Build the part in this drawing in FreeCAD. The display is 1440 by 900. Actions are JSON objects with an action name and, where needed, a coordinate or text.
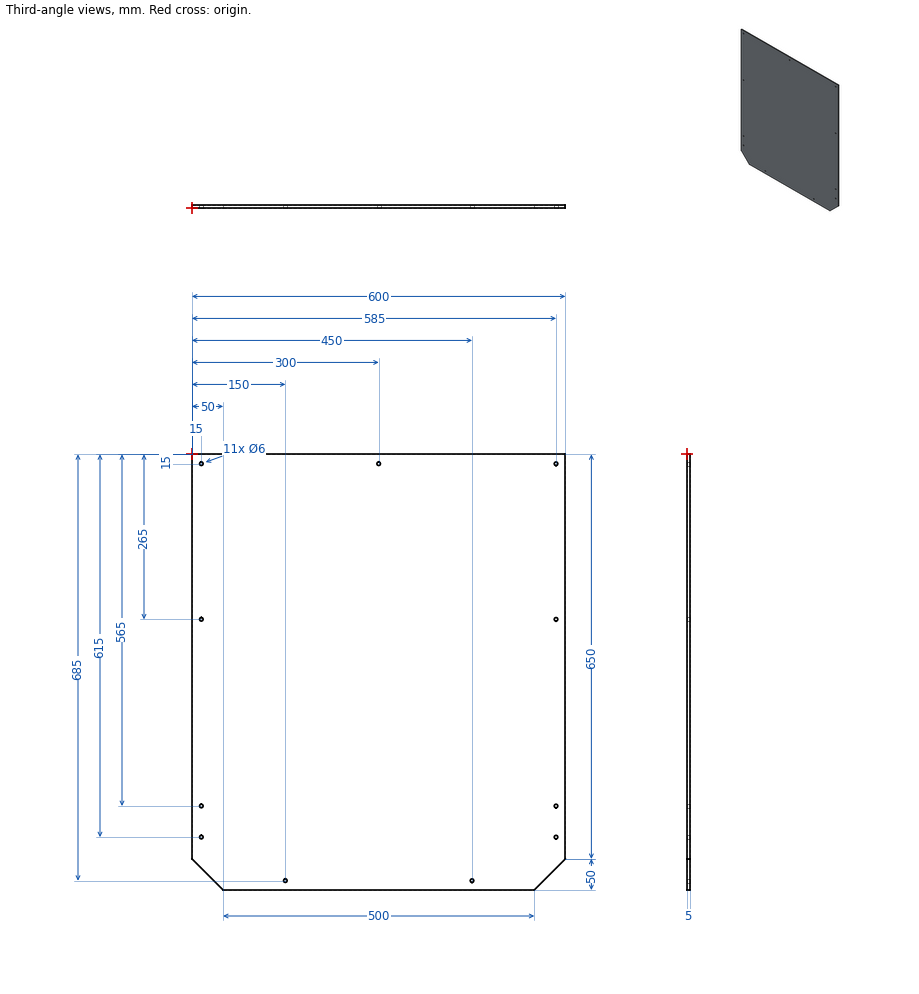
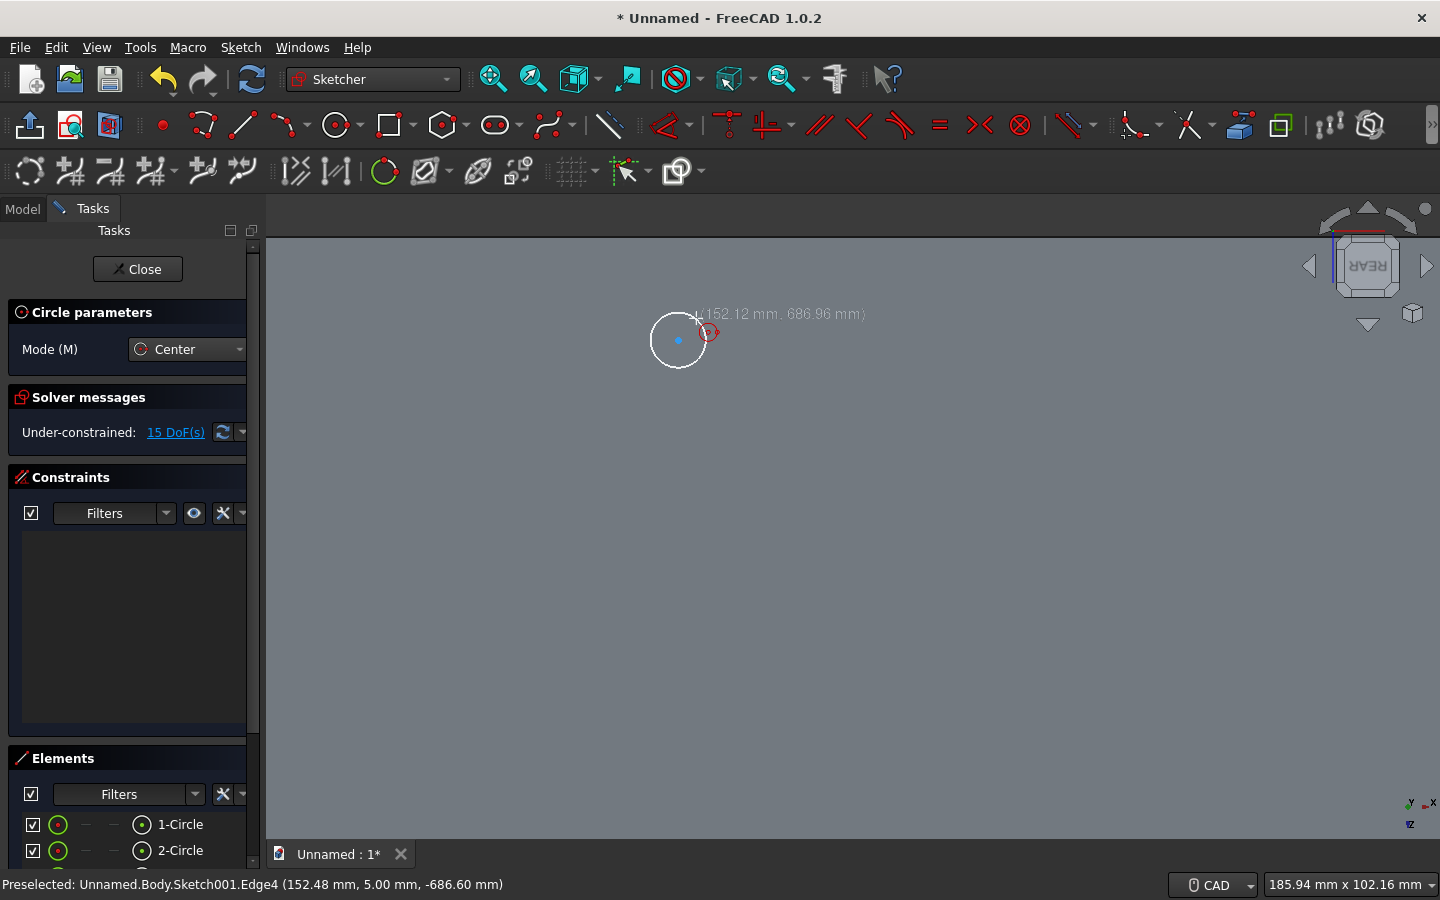
{"action": "scroll", "coordinate": [704, 320], "scroll_direction": "down", "scroll_amount": 12}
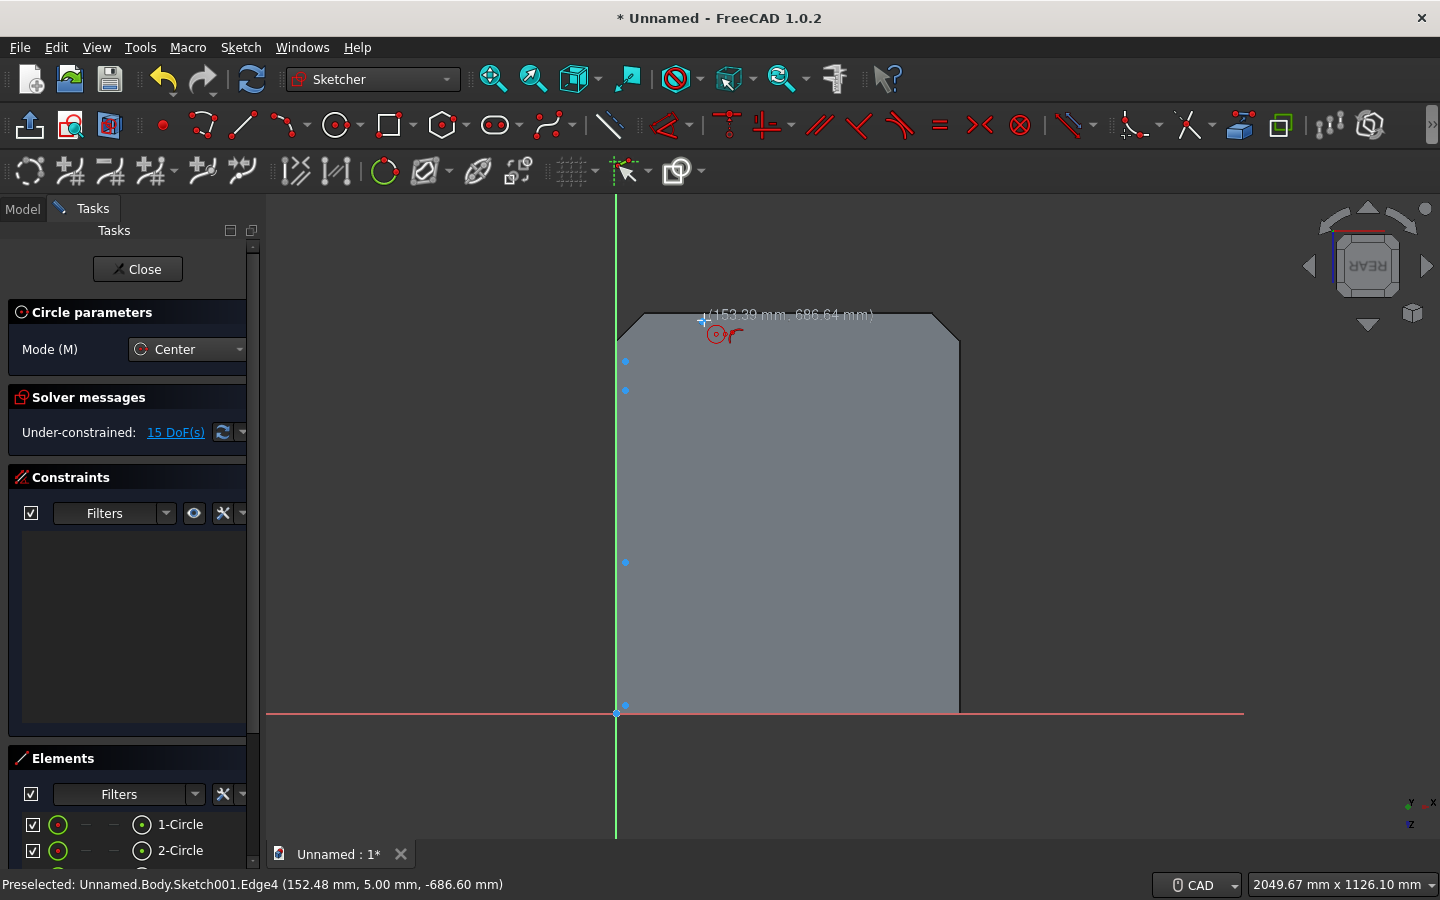
{"action": "scroll", "coordinate": [952, 705], "scroll_direction": "up", "scroll_amount": 13}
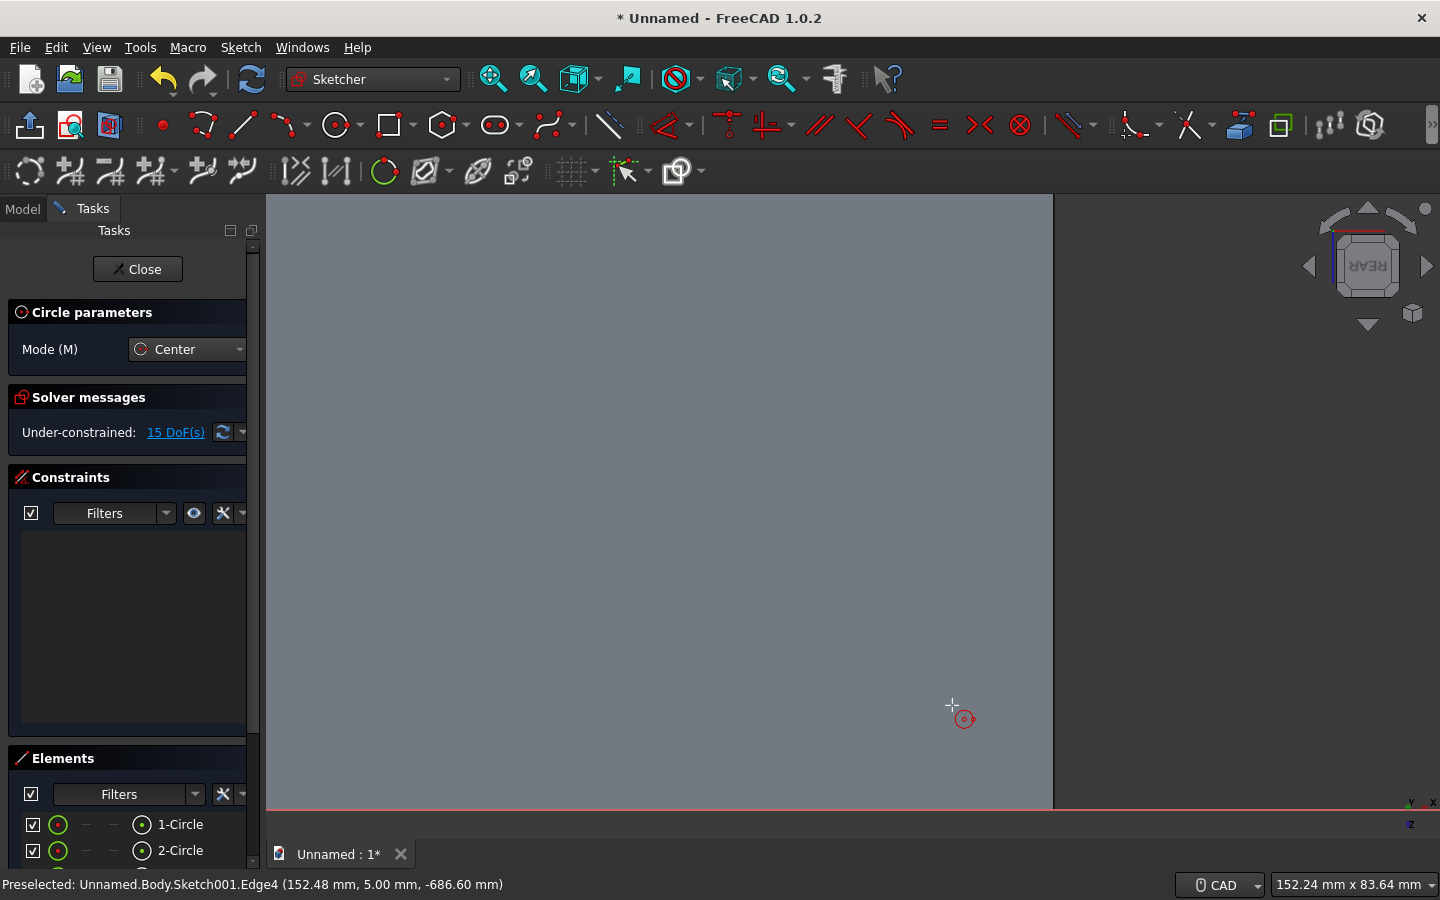
{"action": "scroll", "coordinate": [952, 706], "scroll_direction": "down", "scroll_amount": 13}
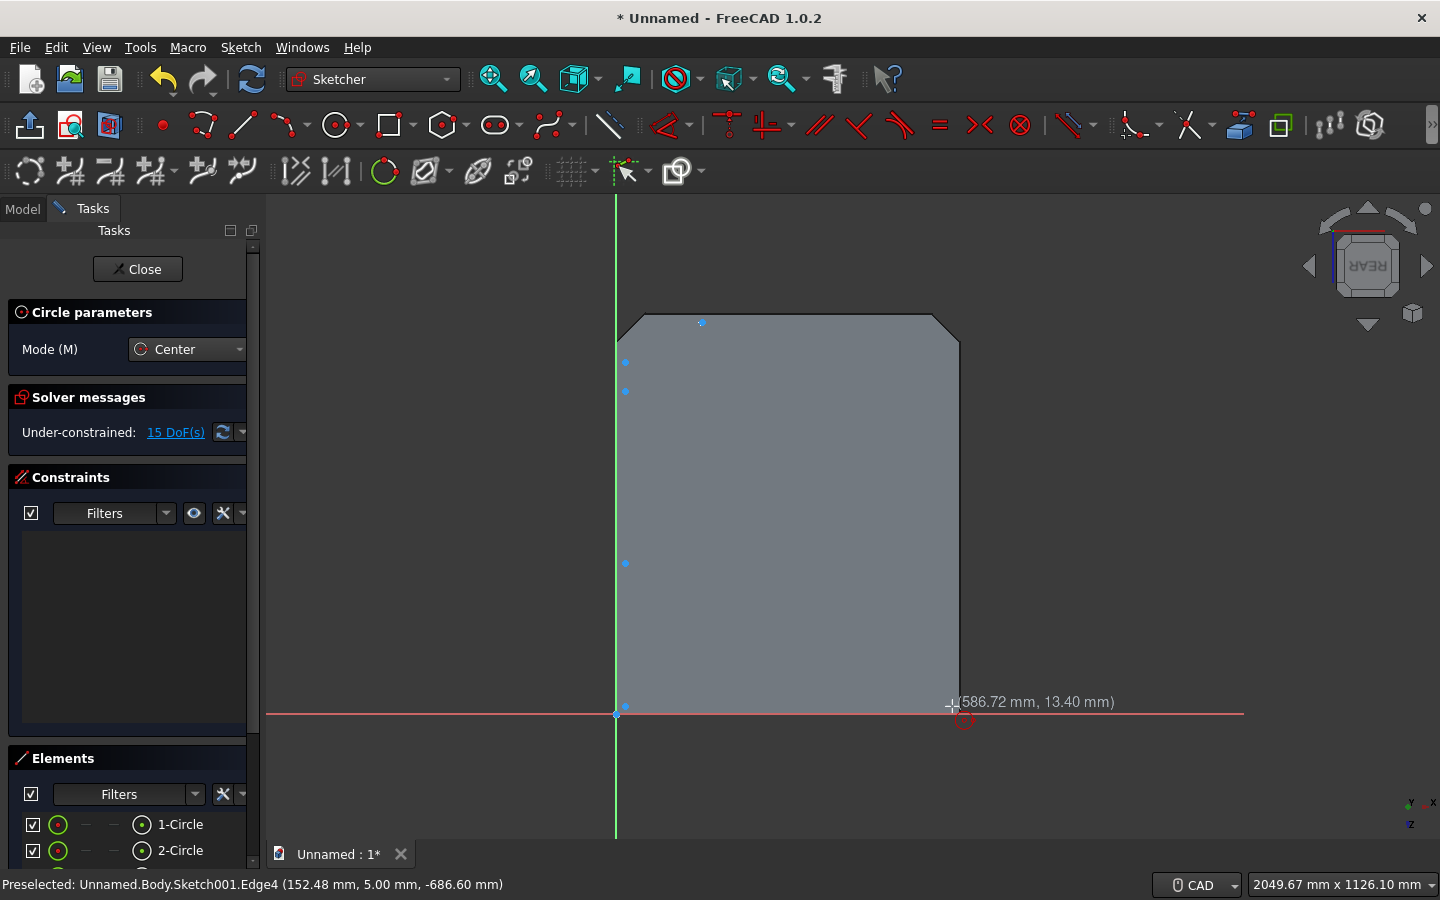
{"action": "scroll", "coordinate": [952, 706], "scroll_direction": "up", "scroll_amount": 4}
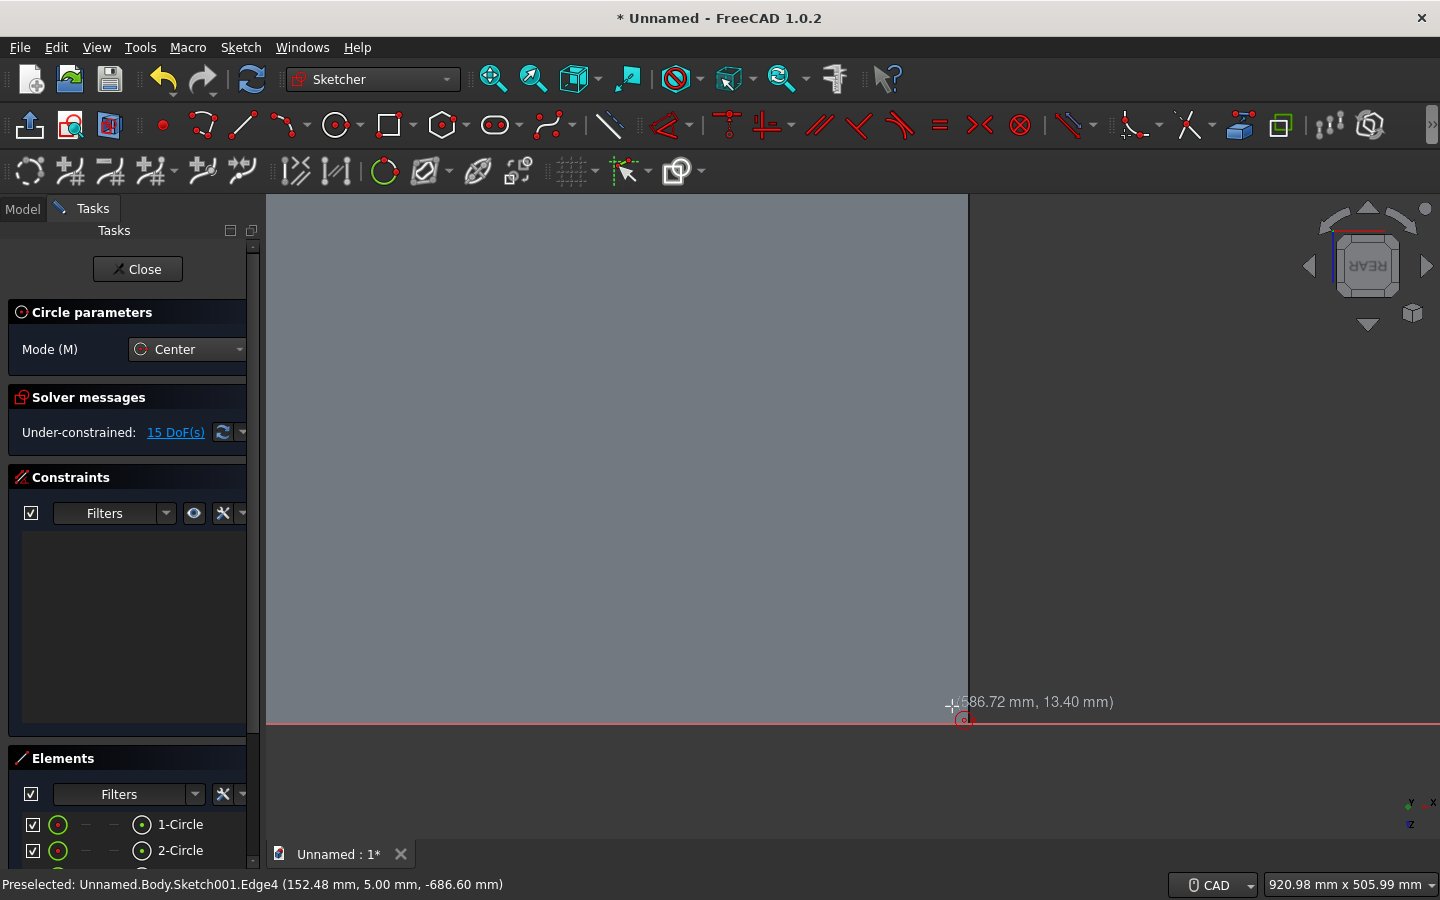
{"action": "left_click", "coordinate": [950, 705]}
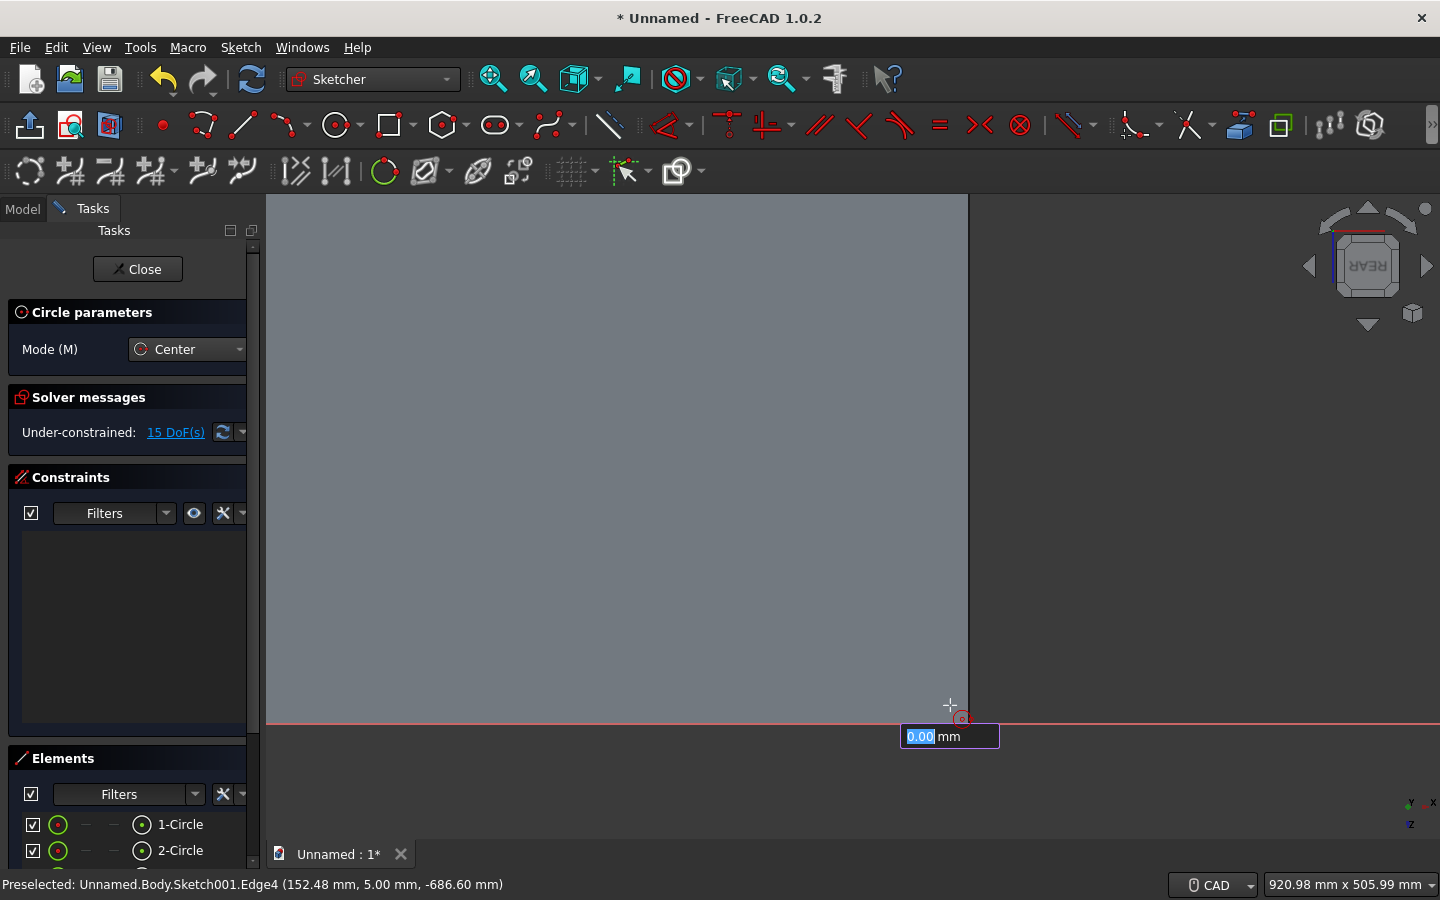
{"action": "scroll", "coordinate": [953, 702], "scroll_direction": "up", "scroll_amount": 8}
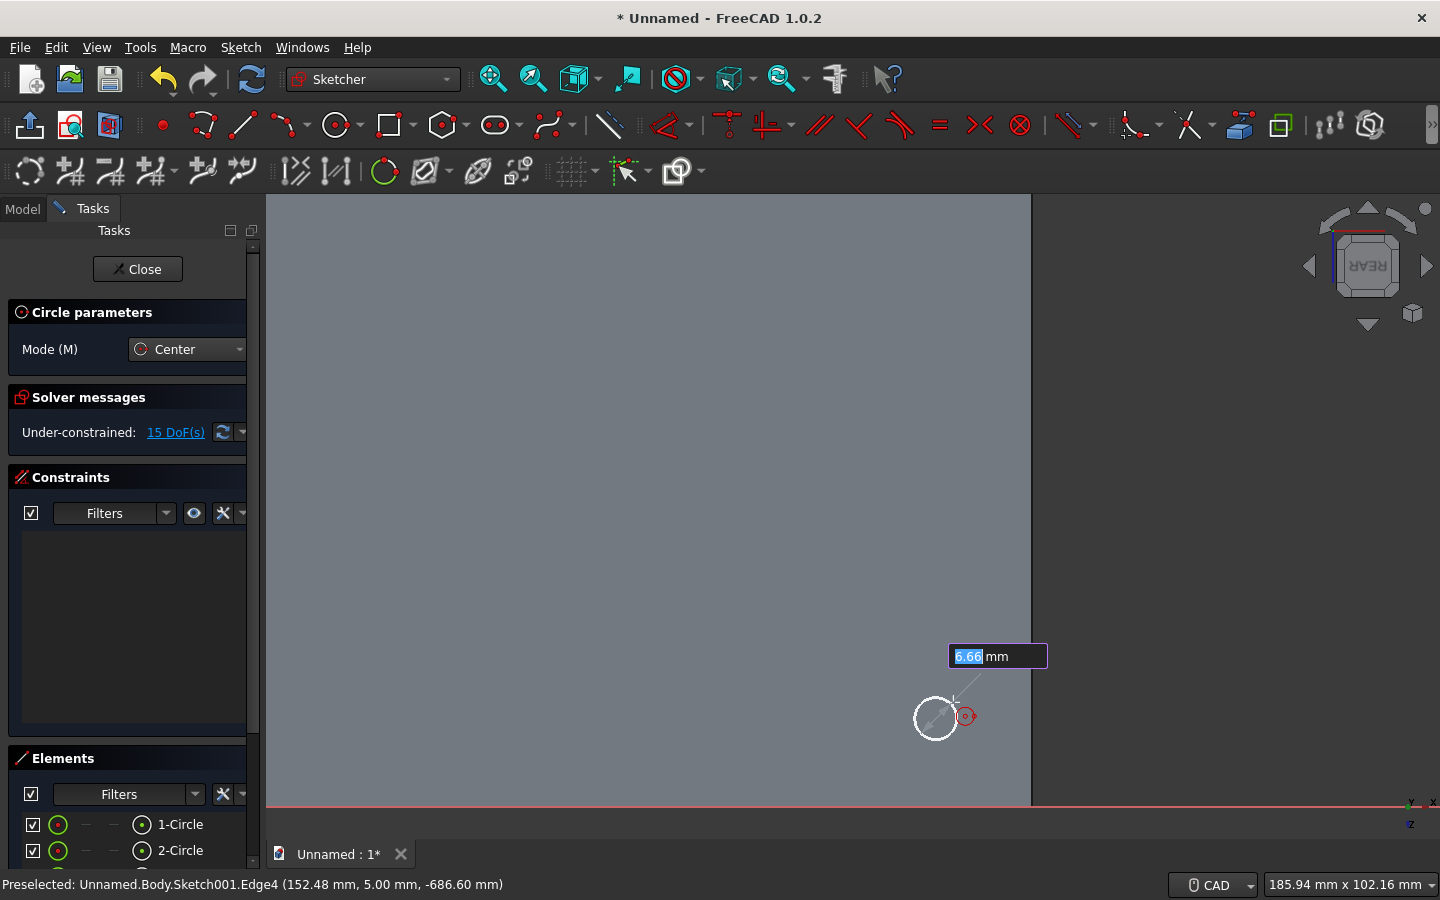
{"action": "left_click", "coordinate": [951, 699]}